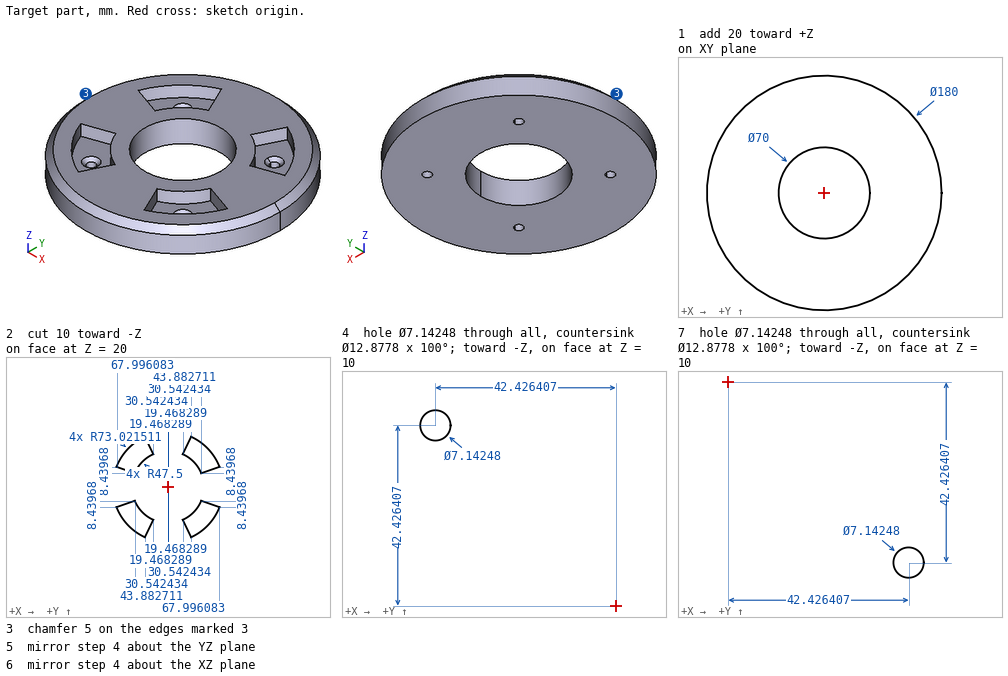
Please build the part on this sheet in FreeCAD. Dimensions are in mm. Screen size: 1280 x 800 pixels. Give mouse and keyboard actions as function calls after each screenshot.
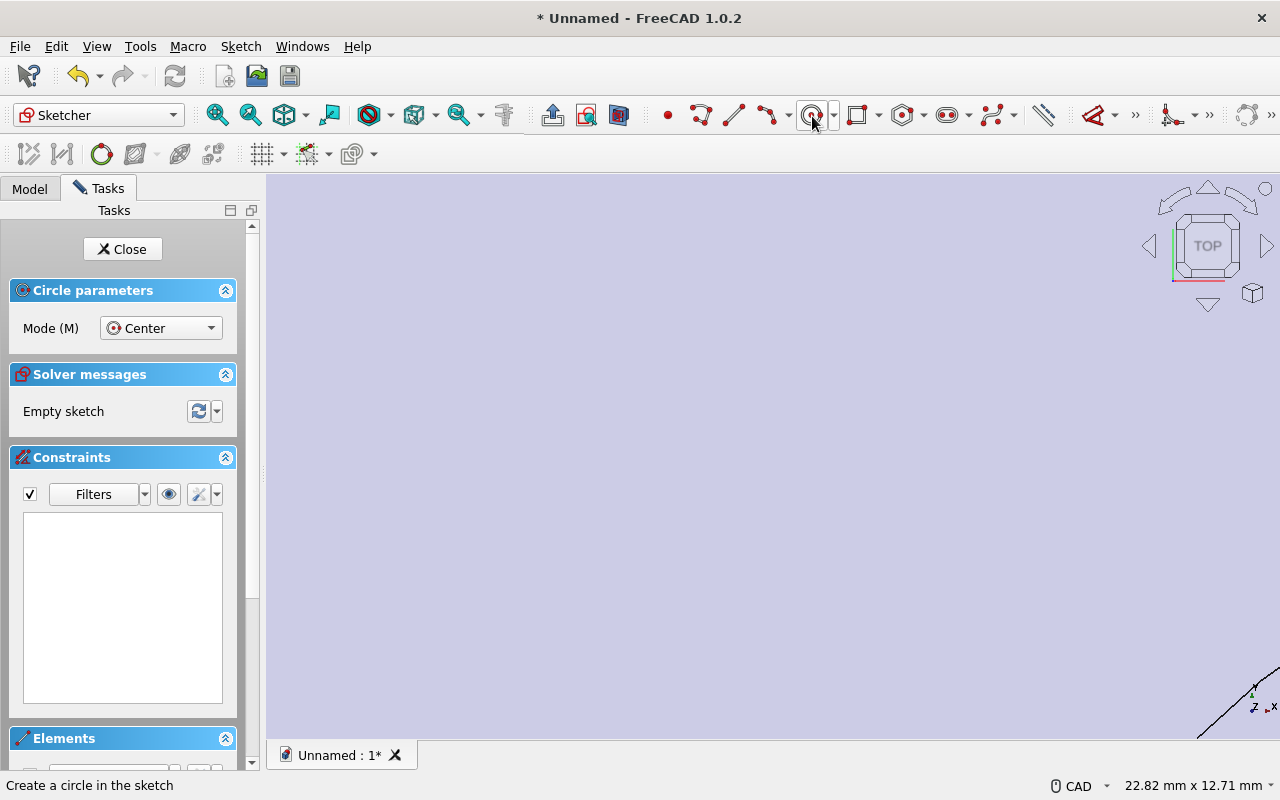
click(693, 445)
move(805, 332)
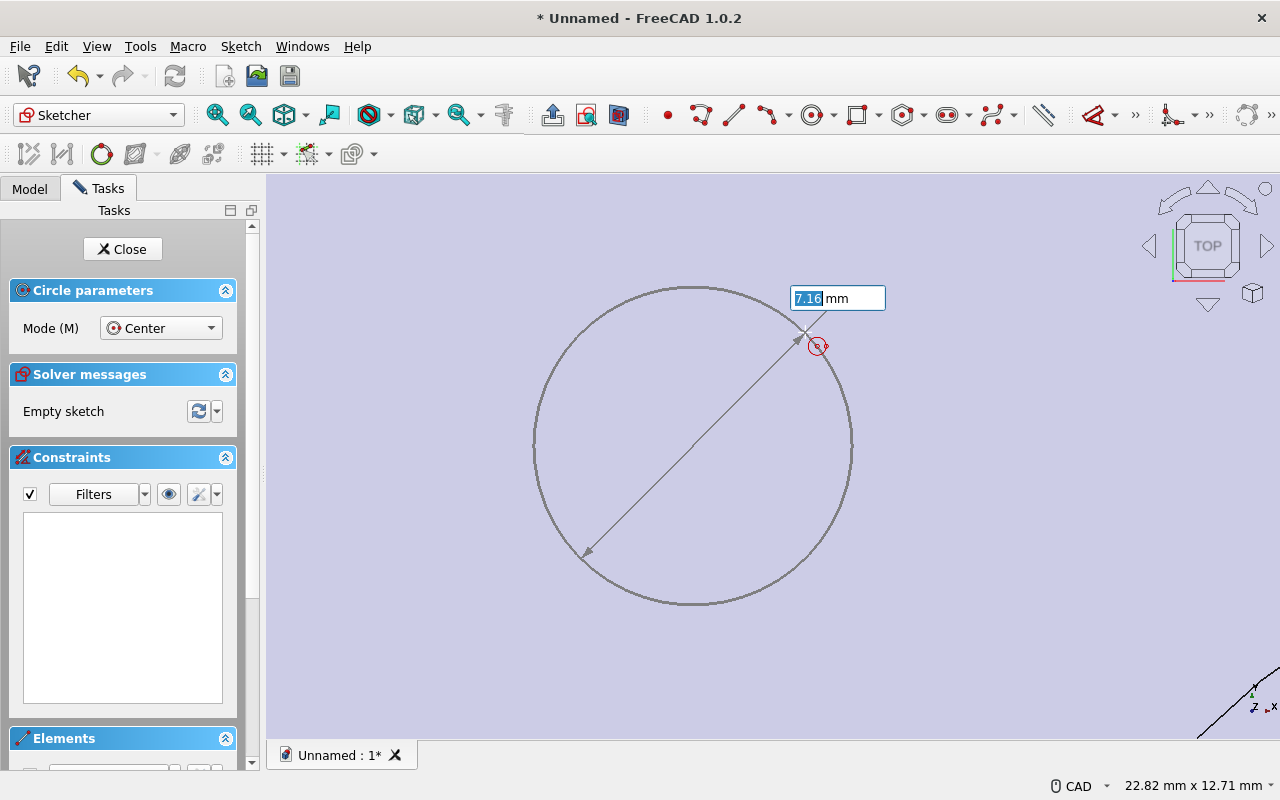
text(7.14248)
key(Return)
key(Escape)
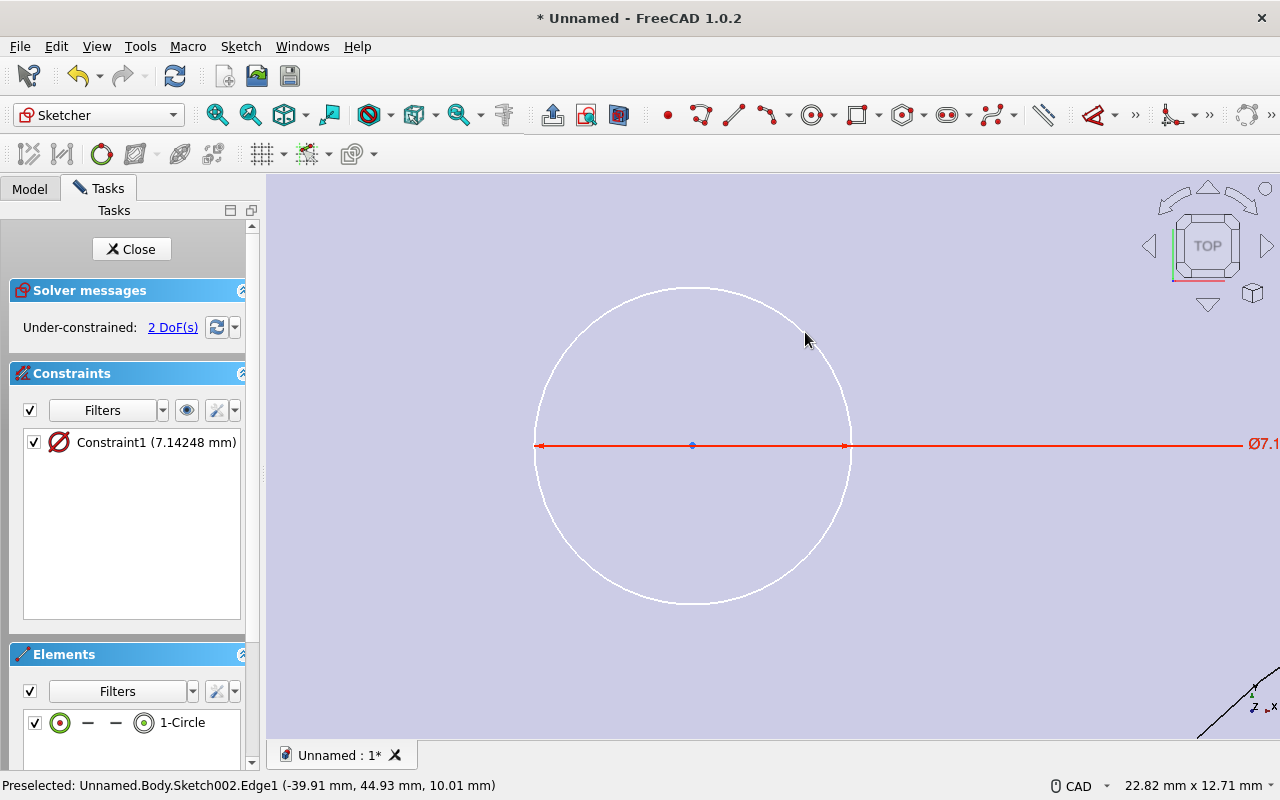
key(d)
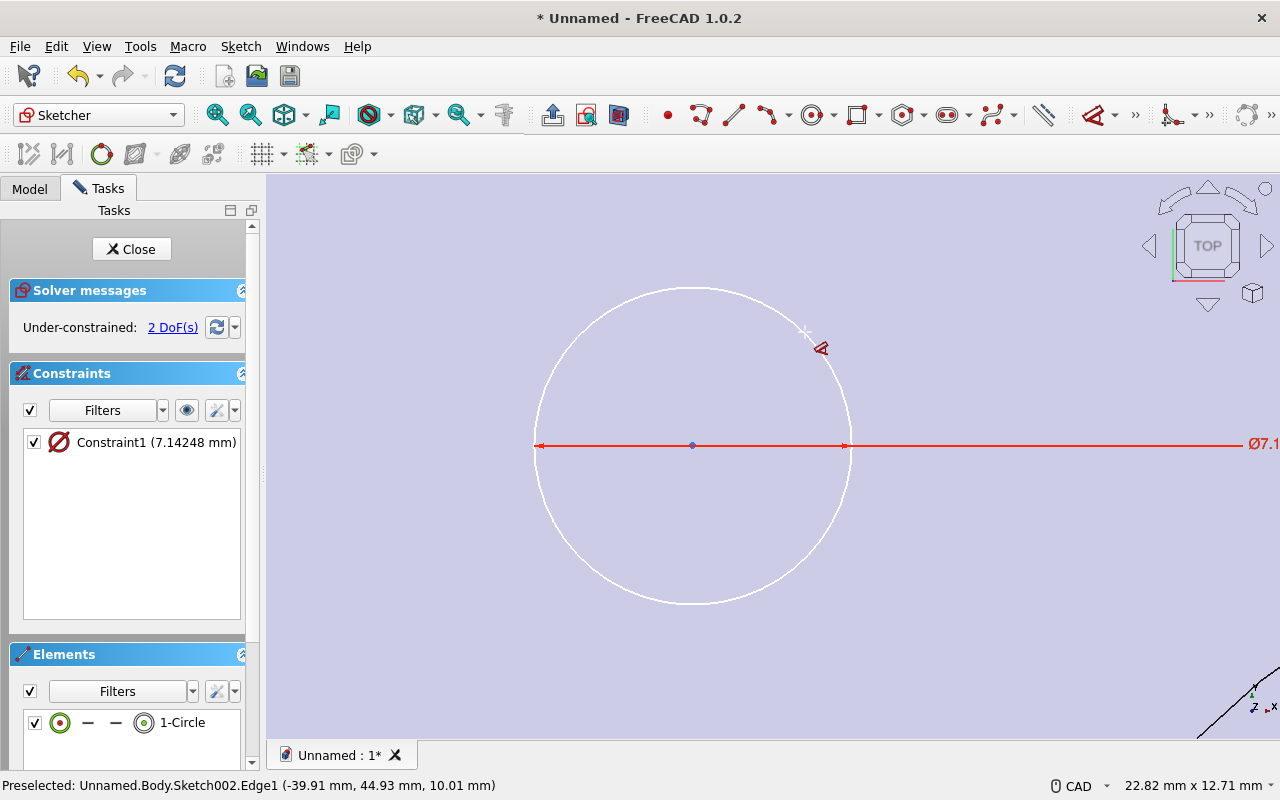
click(693, 446)
click(904, 412)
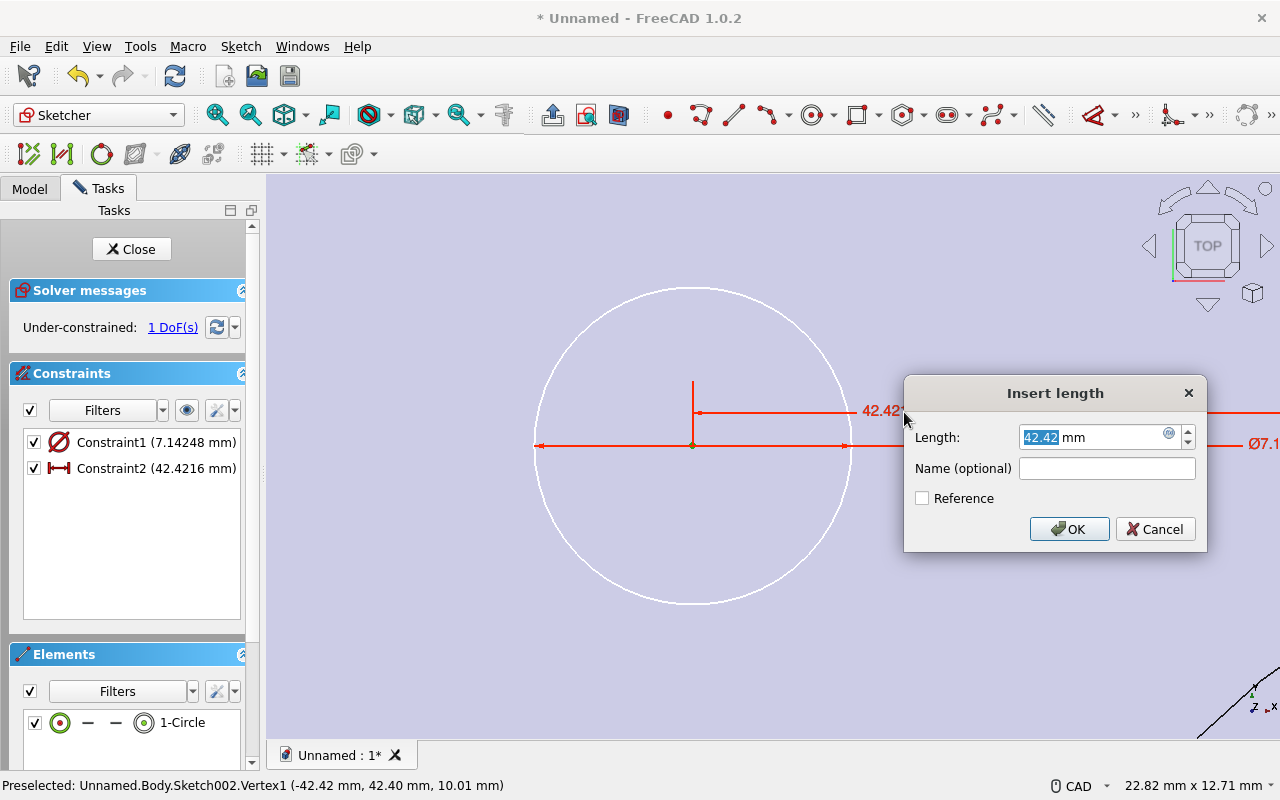
text(42.426407)
key(Return)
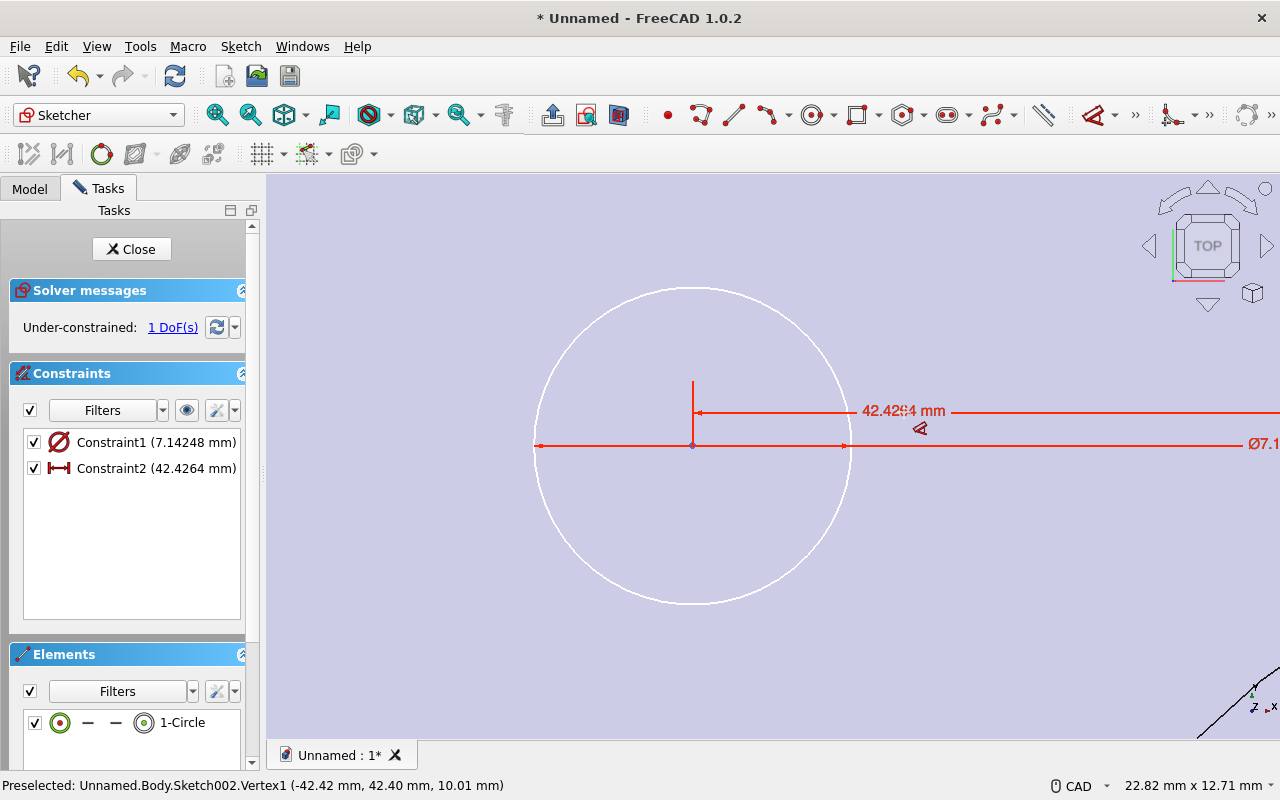
click(693, 446)
click(659, 578)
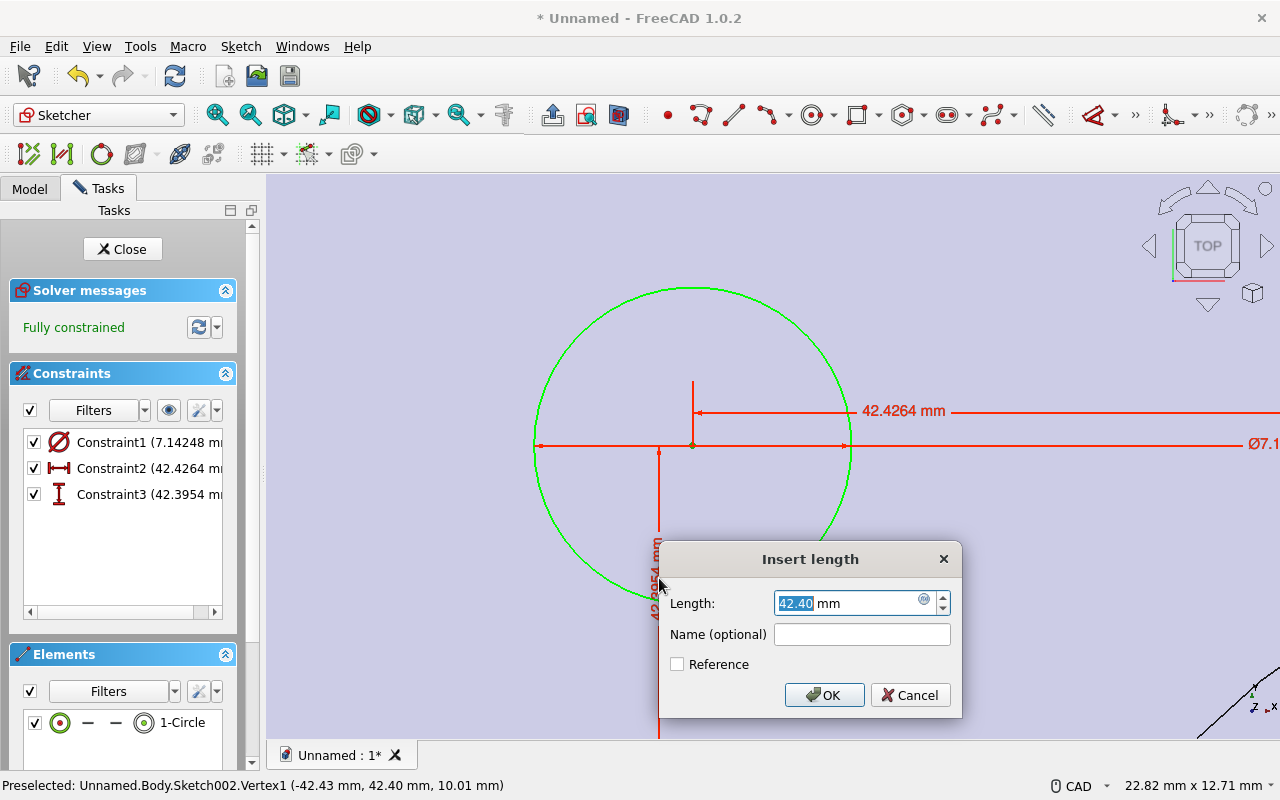
text(42.426407)
key(Return)
key(Escape)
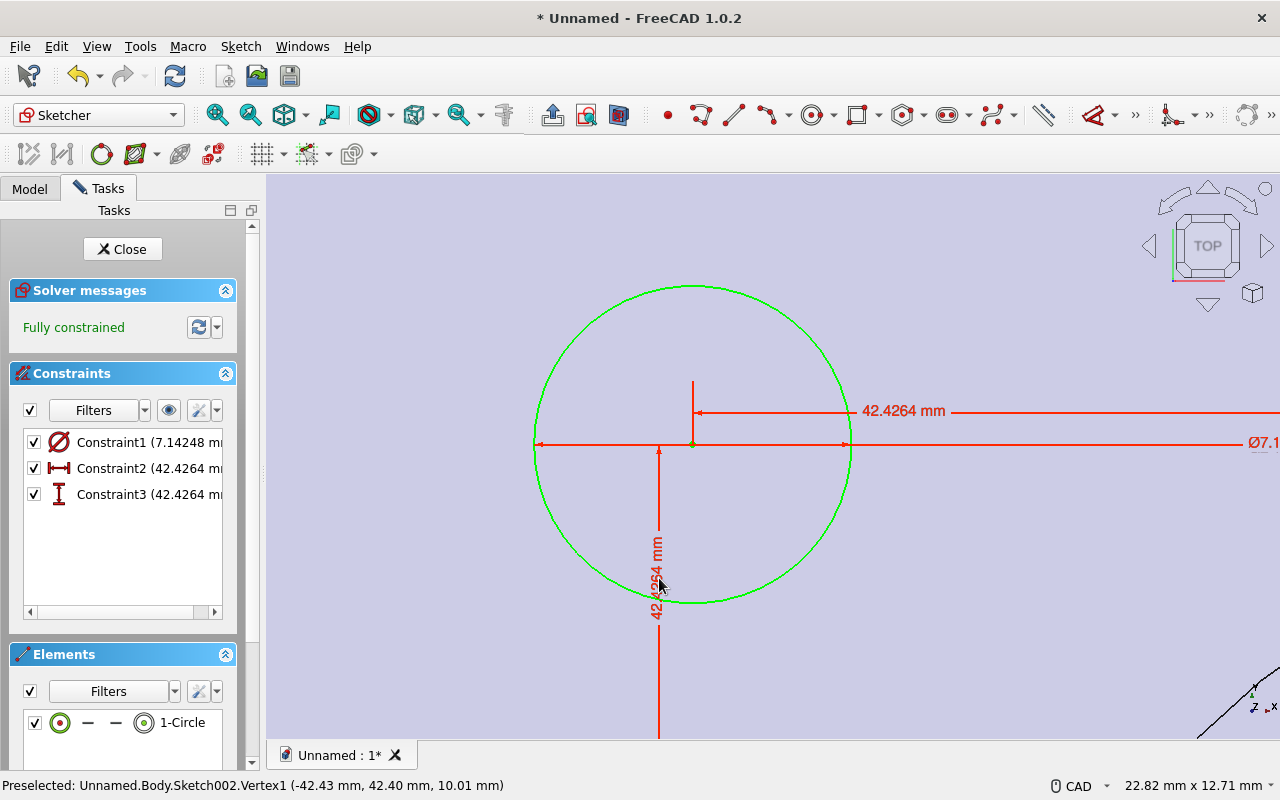
click(123, 249)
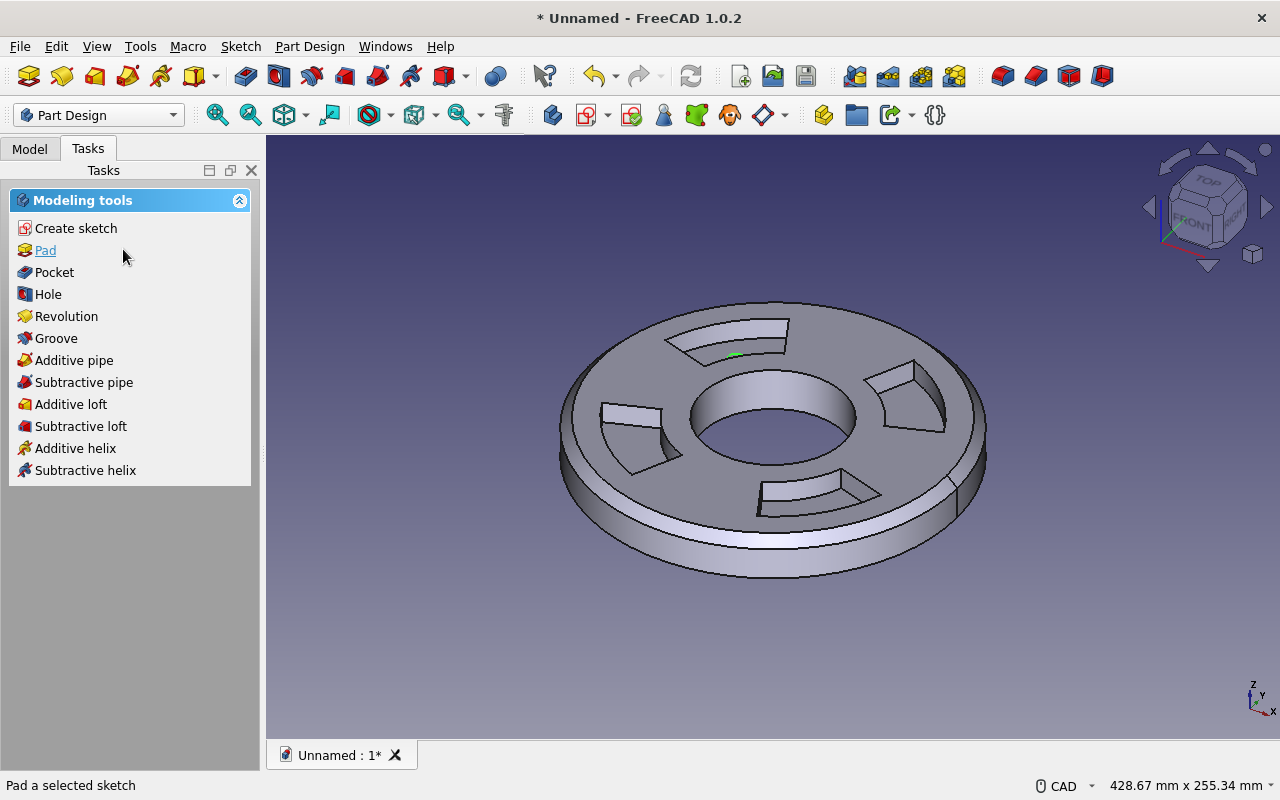
click(279, 76)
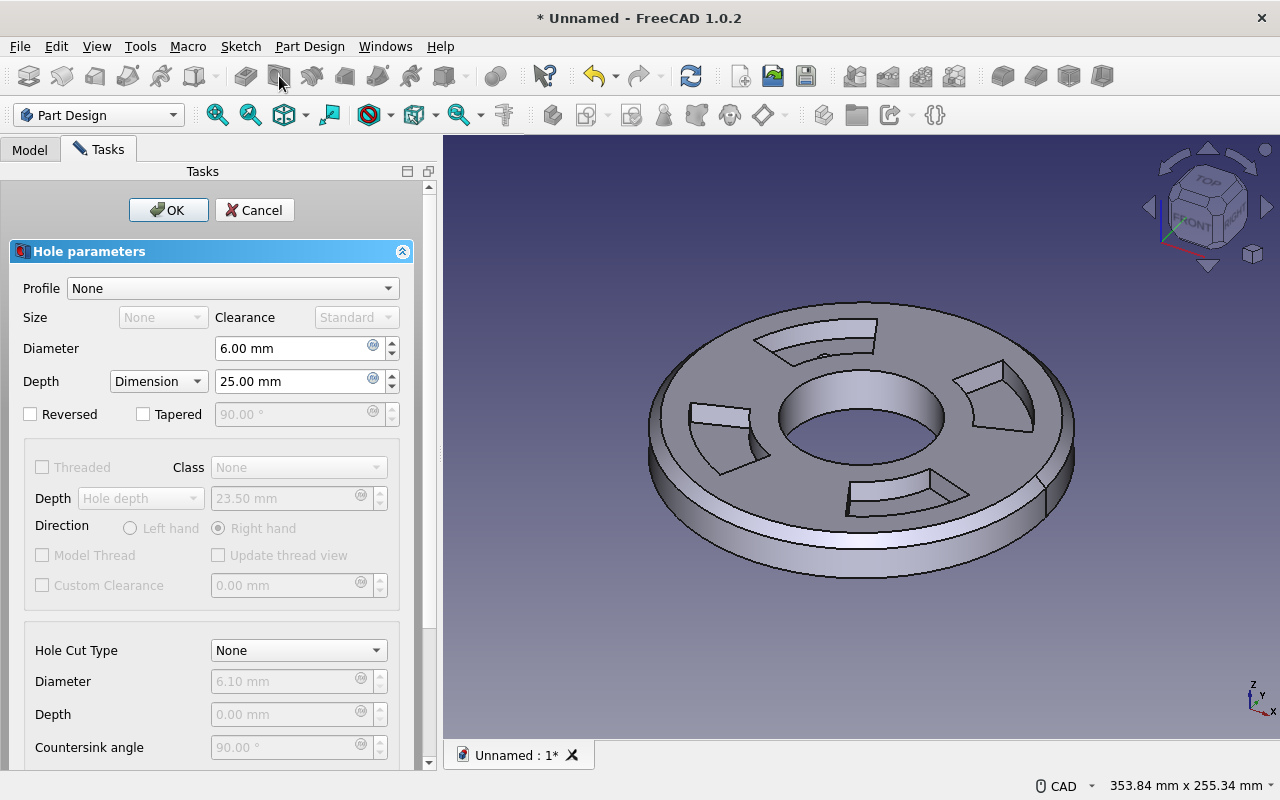
triple_click(300, 348)